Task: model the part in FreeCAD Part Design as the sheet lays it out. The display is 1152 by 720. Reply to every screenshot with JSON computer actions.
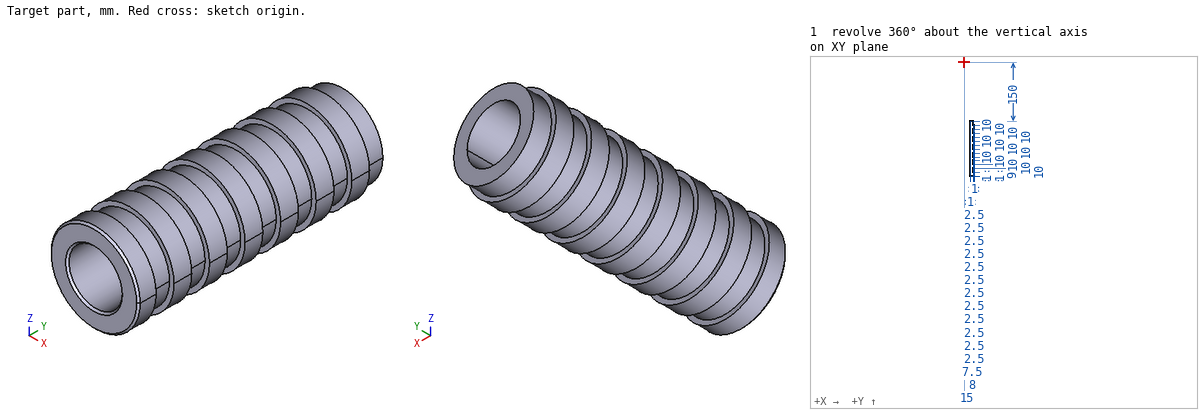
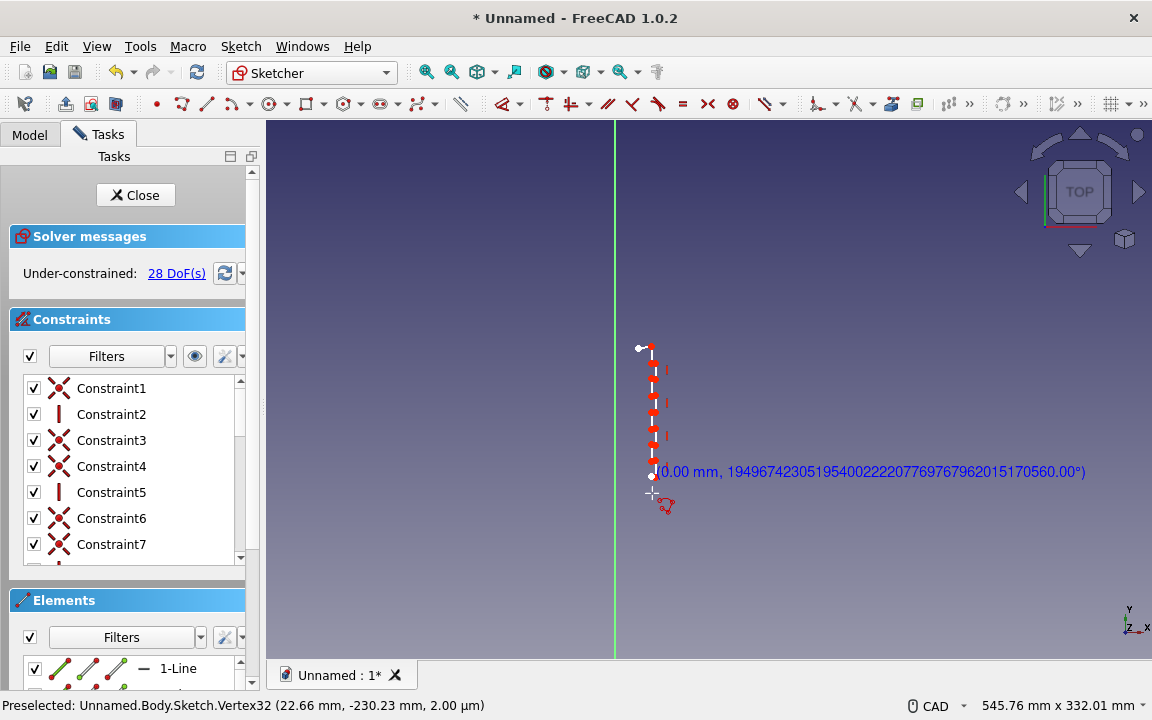
{"action": "left_click", "coordinate": [652, 493]}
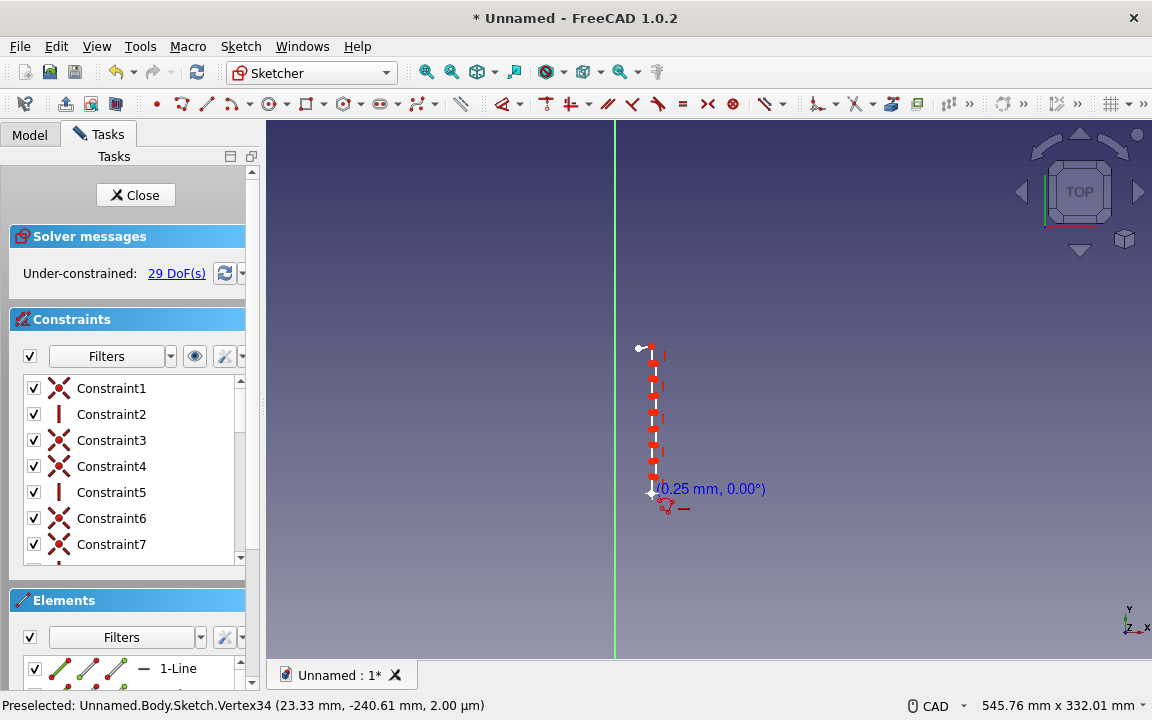
{"action": "scroll", "coordinate": [656, 493], "scroll_direction": "up", "scroll_amount": 7}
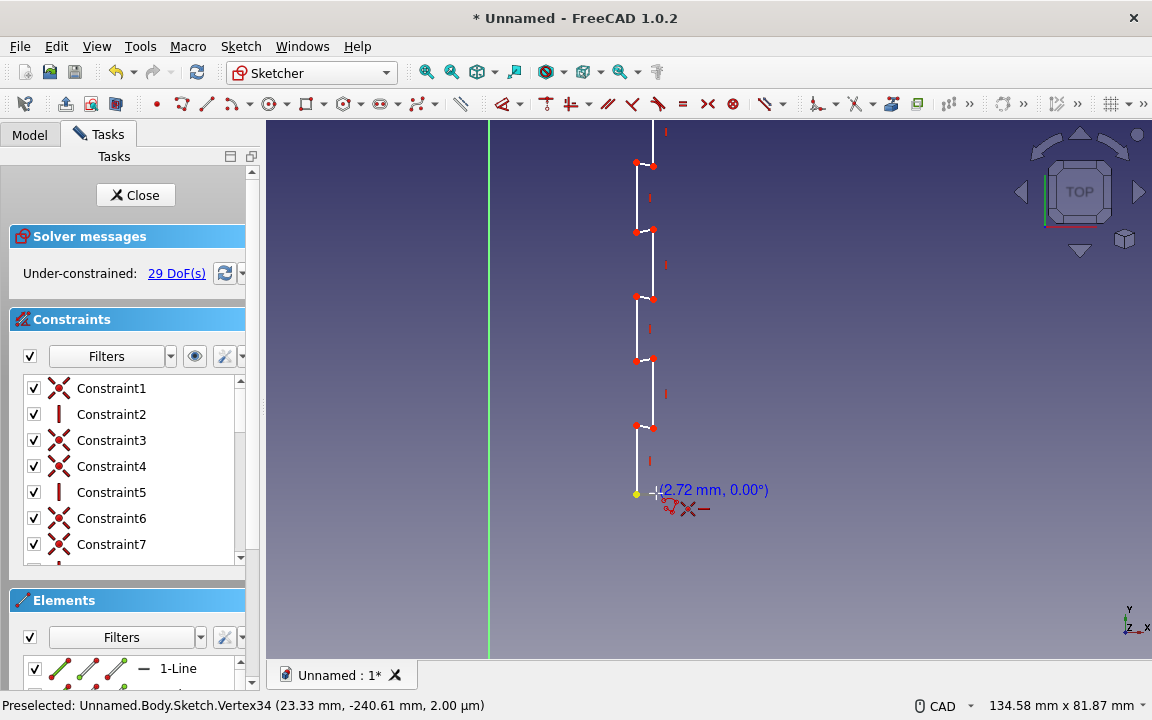
{"action": "left_click", "coordinate": [653, 491]}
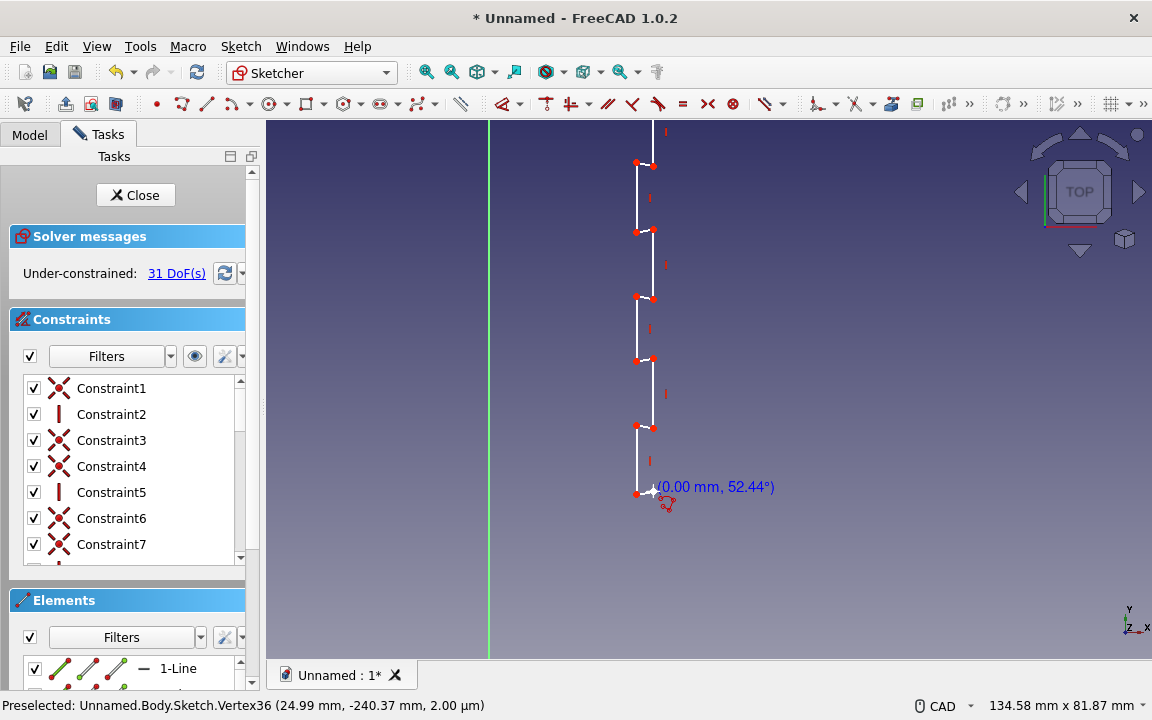
{"action": "scroll", "coordinate": [654, 493], "scroll_direction": "down", "scroll_amount": 9}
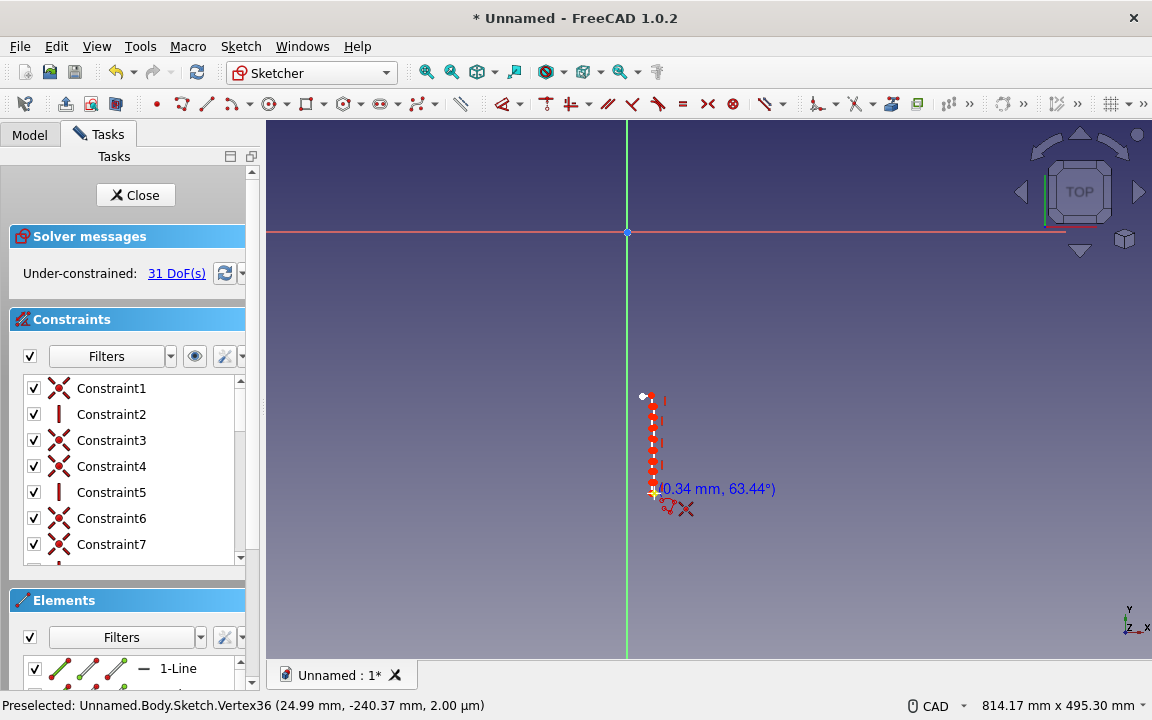
{"action": "scroll", "coordinate": [654, 504], "scroll_direction": "up", "scroll_amount": 2}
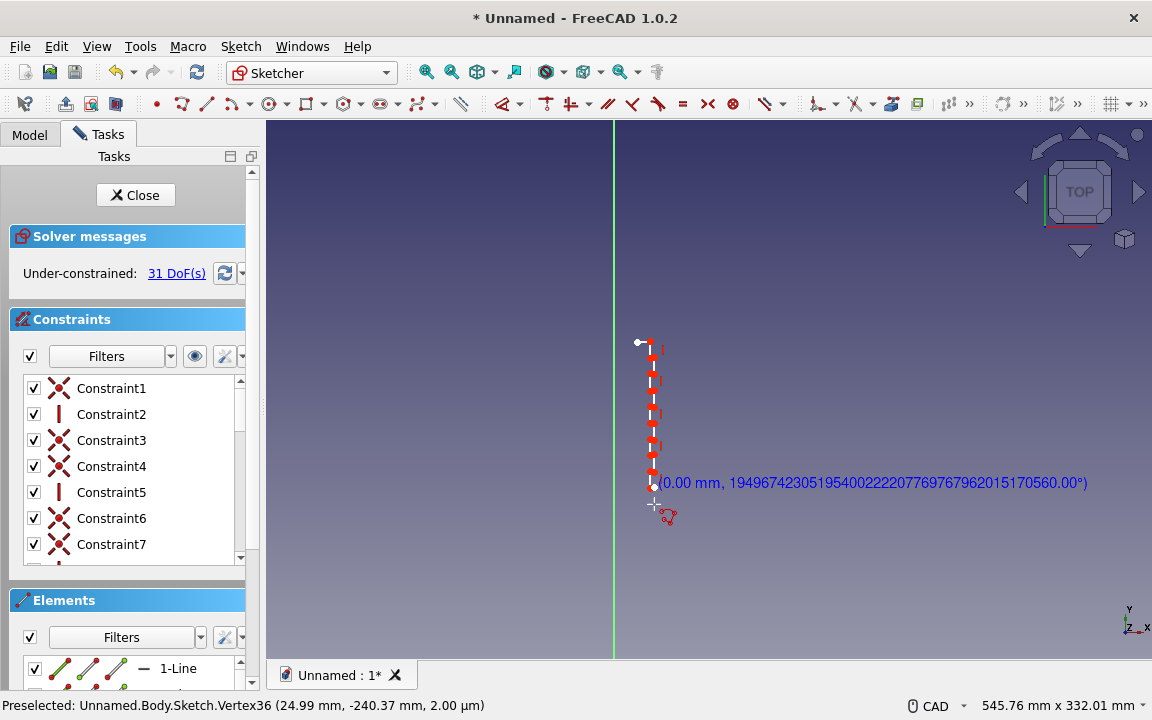
{"action": "left_click", "coordinate": [654, 504]}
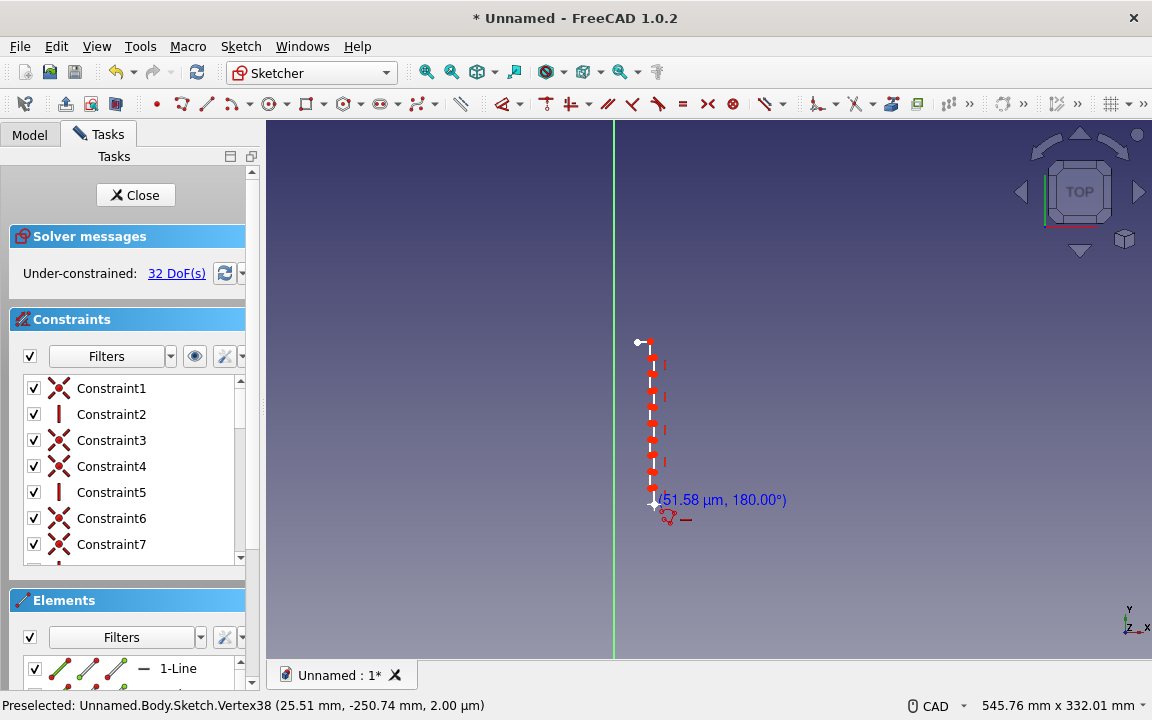
{"action": "scroll", "coordinate": [650, 504], "scroll_direction": "up", "scroll_amount": 7}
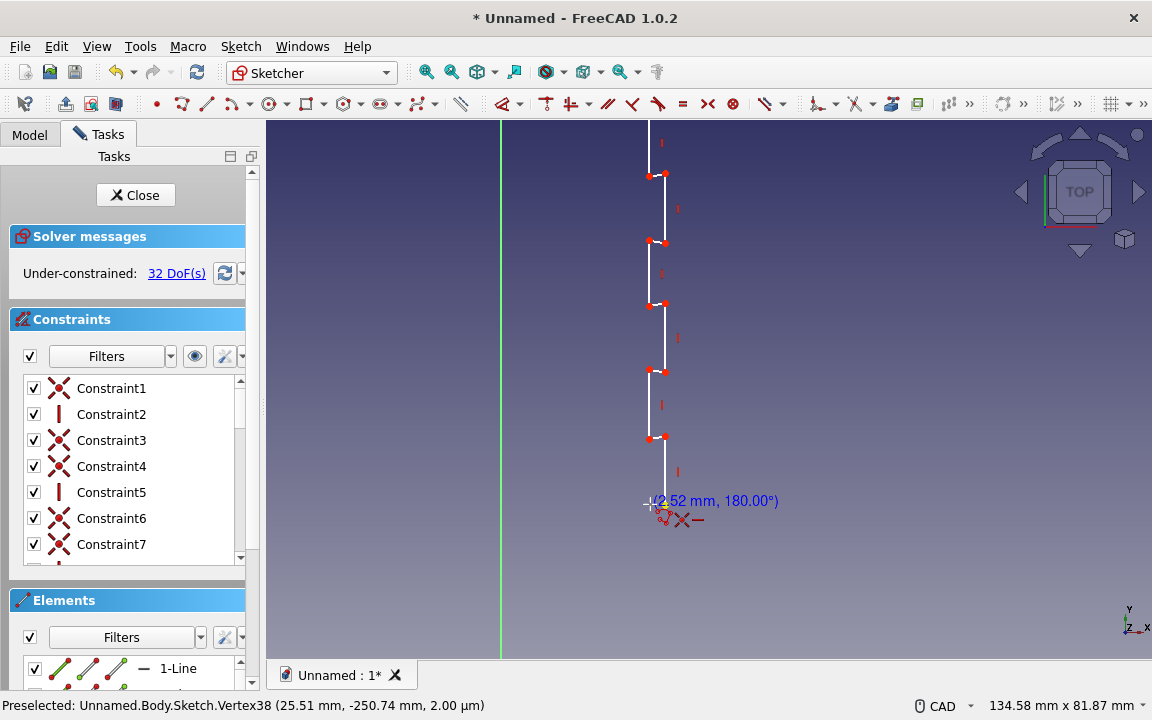
{"action": "left_click", "coordinate": [649, 502]}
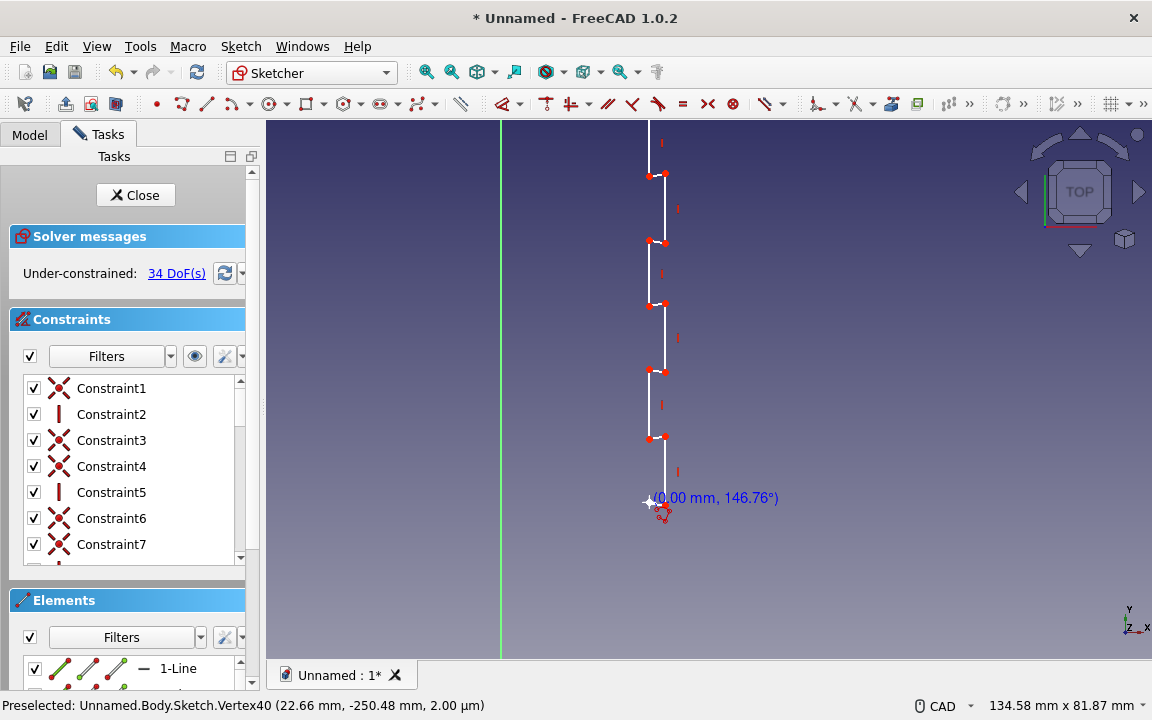
{"action": "scroll", "coordinate": [652, 504], "scroll_direction": "down", "scroll_amount": 9}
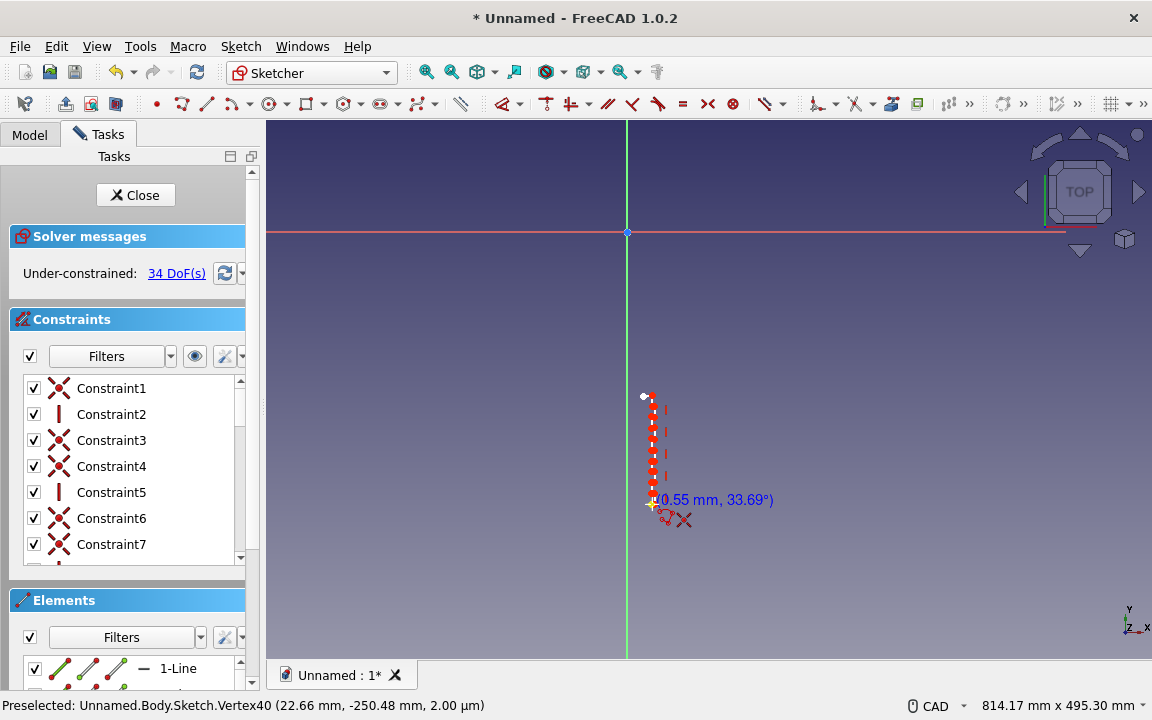
{"action": "scroll", "coordinate": [652, 515], "scroll_direction": "up", "scroll_amount": 2}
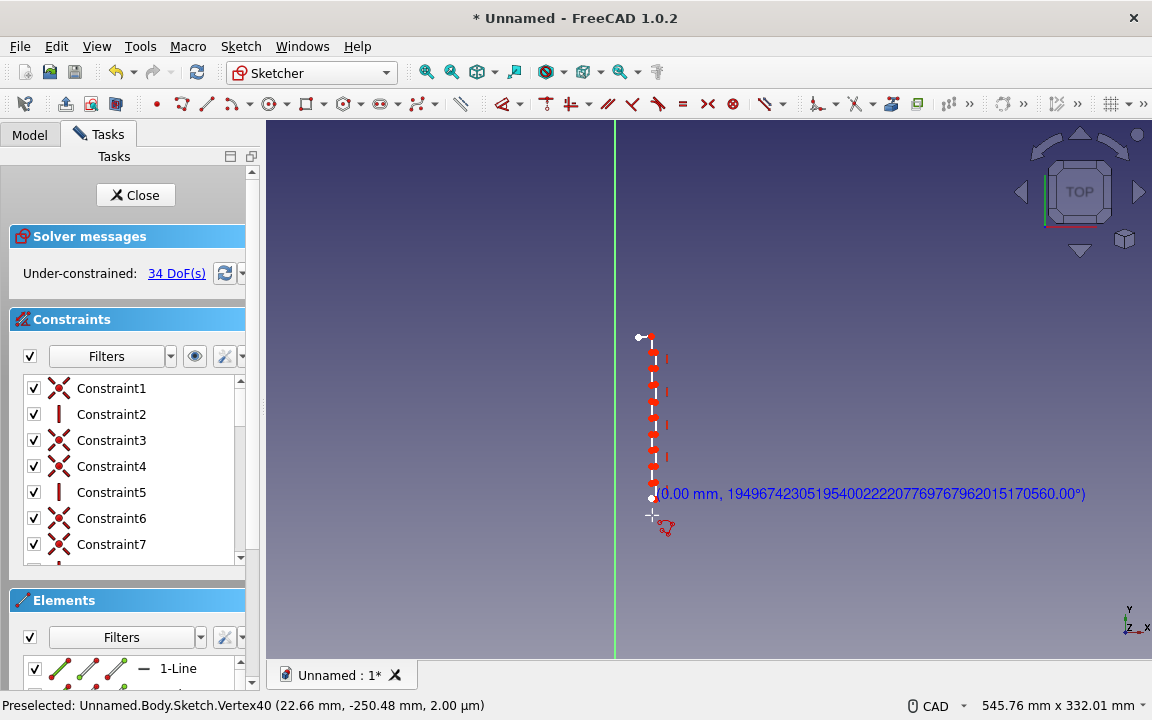
{"action": "left_click", "coordinate": [652, 515]}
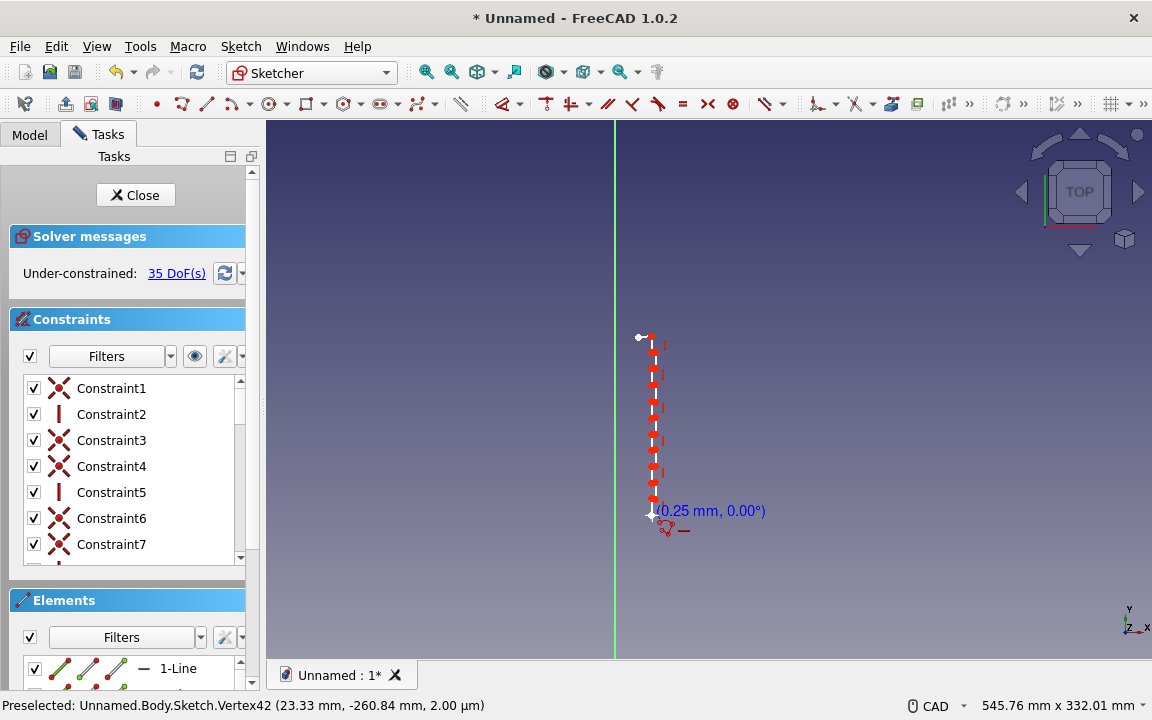
{"action": "scroll", "coordinate": [656, 515], "scroll_direction": "up", "scroll_amount": 7}